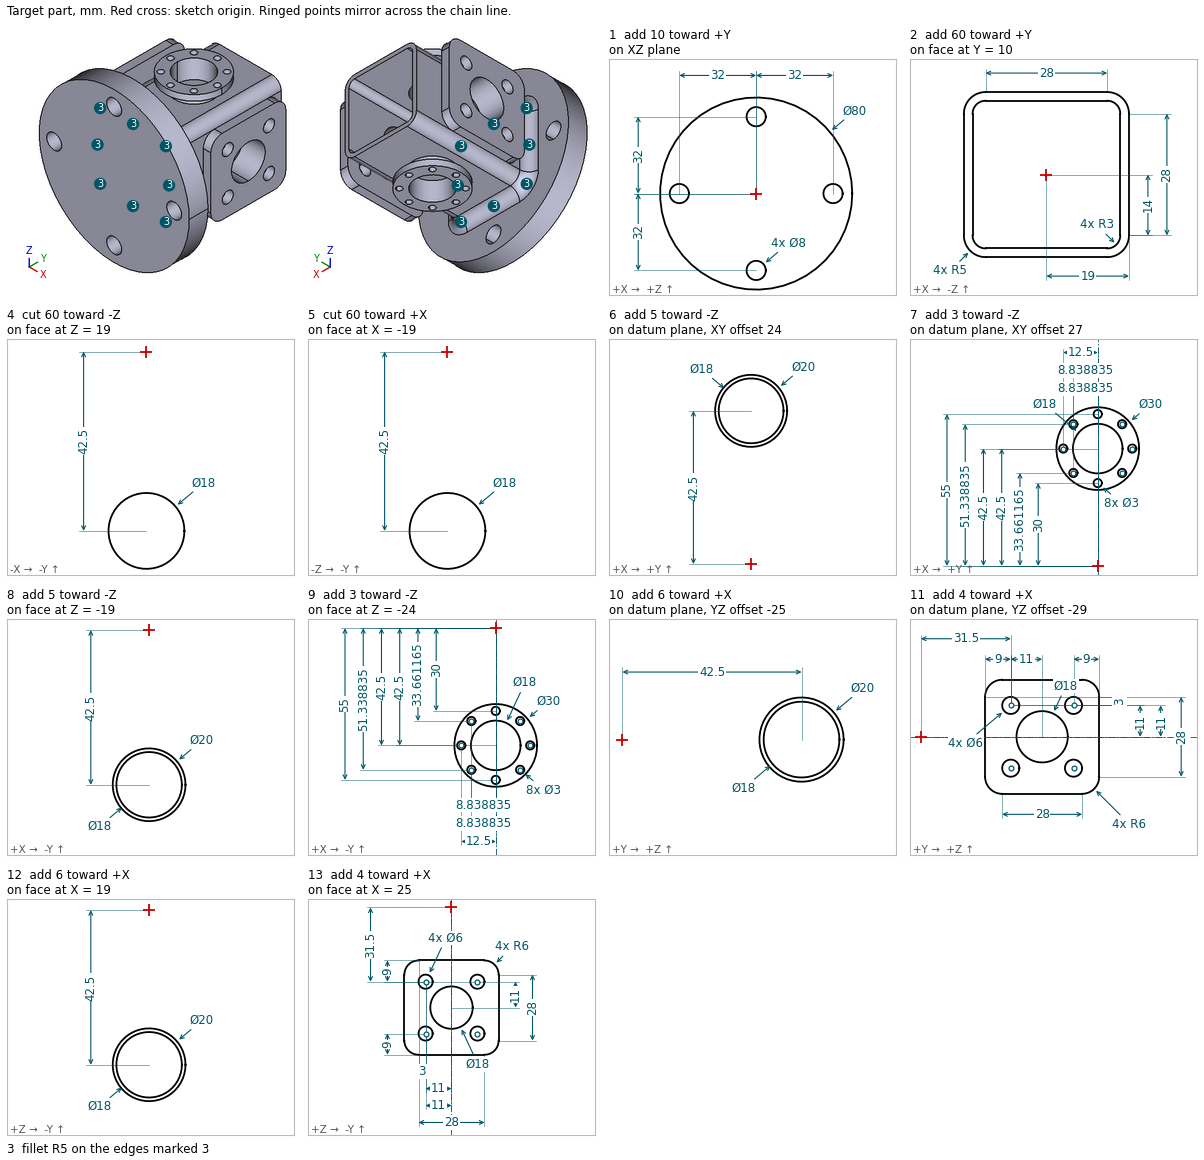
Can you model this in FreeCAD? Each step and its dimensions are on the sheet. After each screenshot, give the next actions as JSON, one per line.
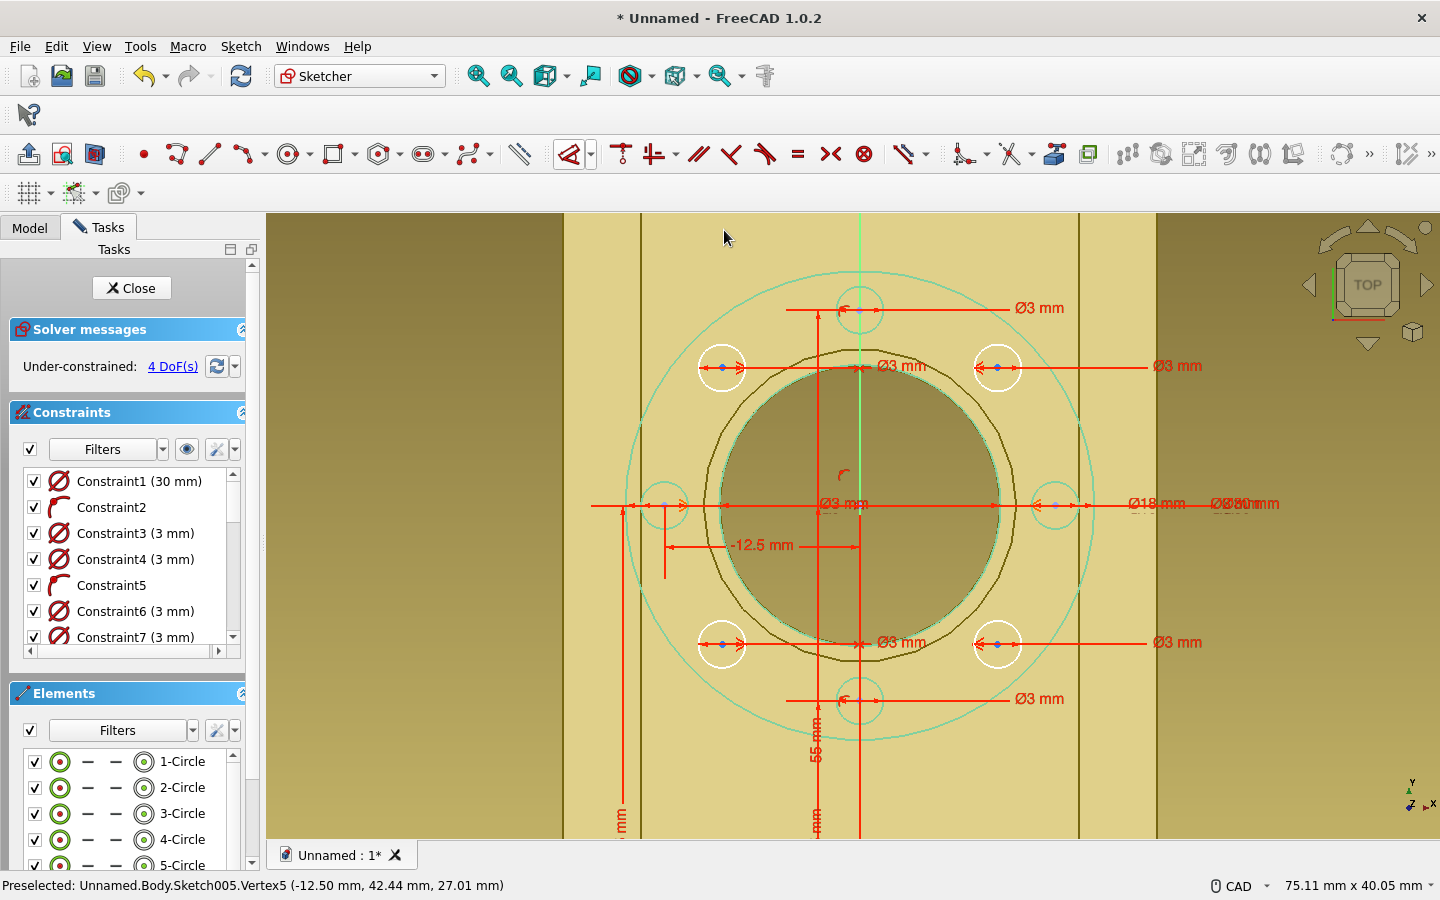
{"action": "left_click", "coordinate": [722, 644]}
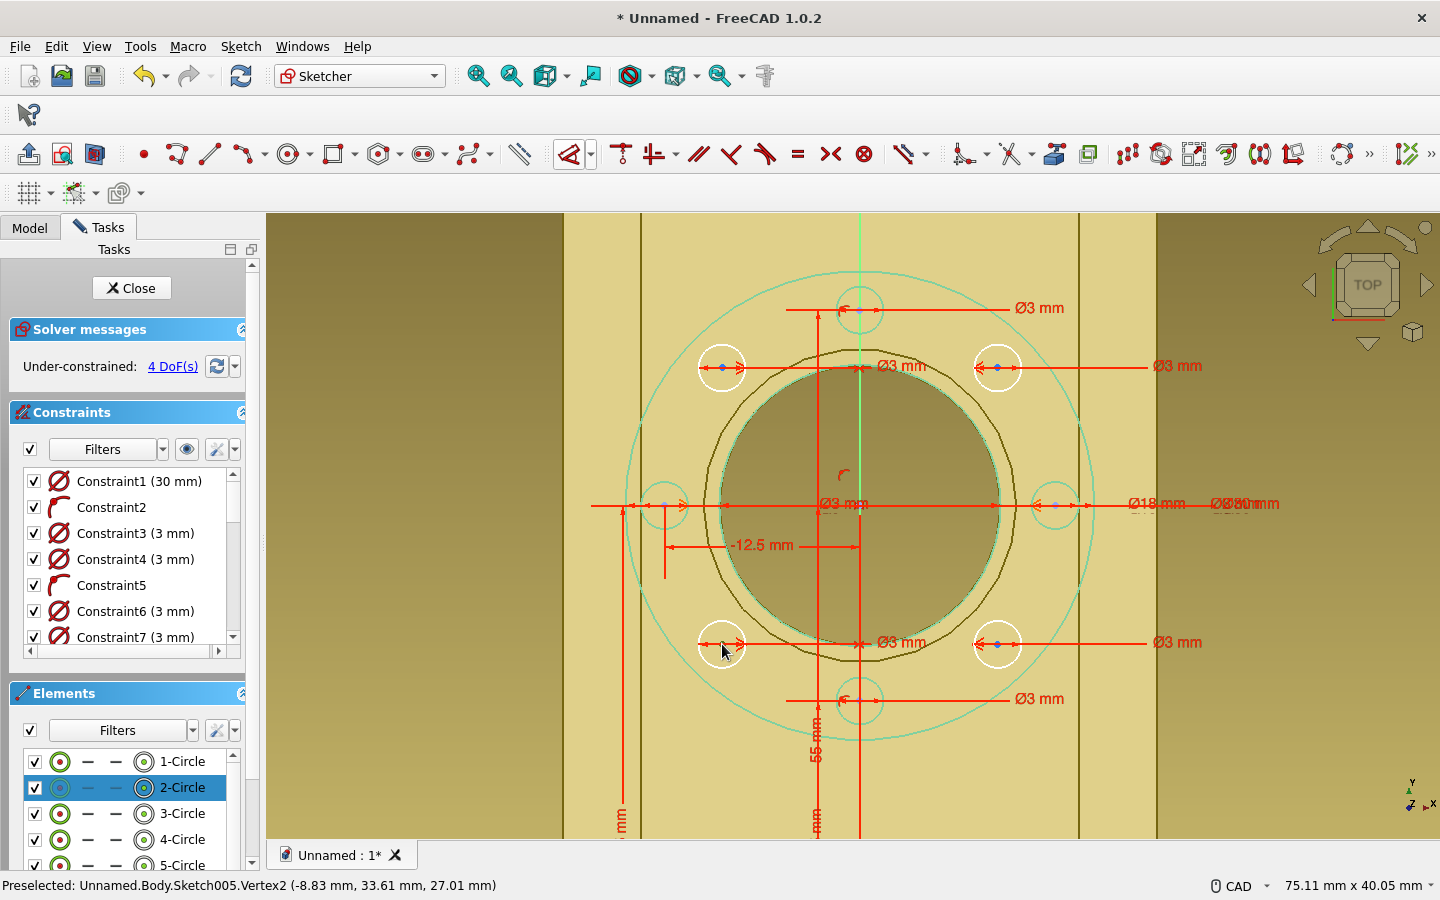
{"action": "key", "text": "l"}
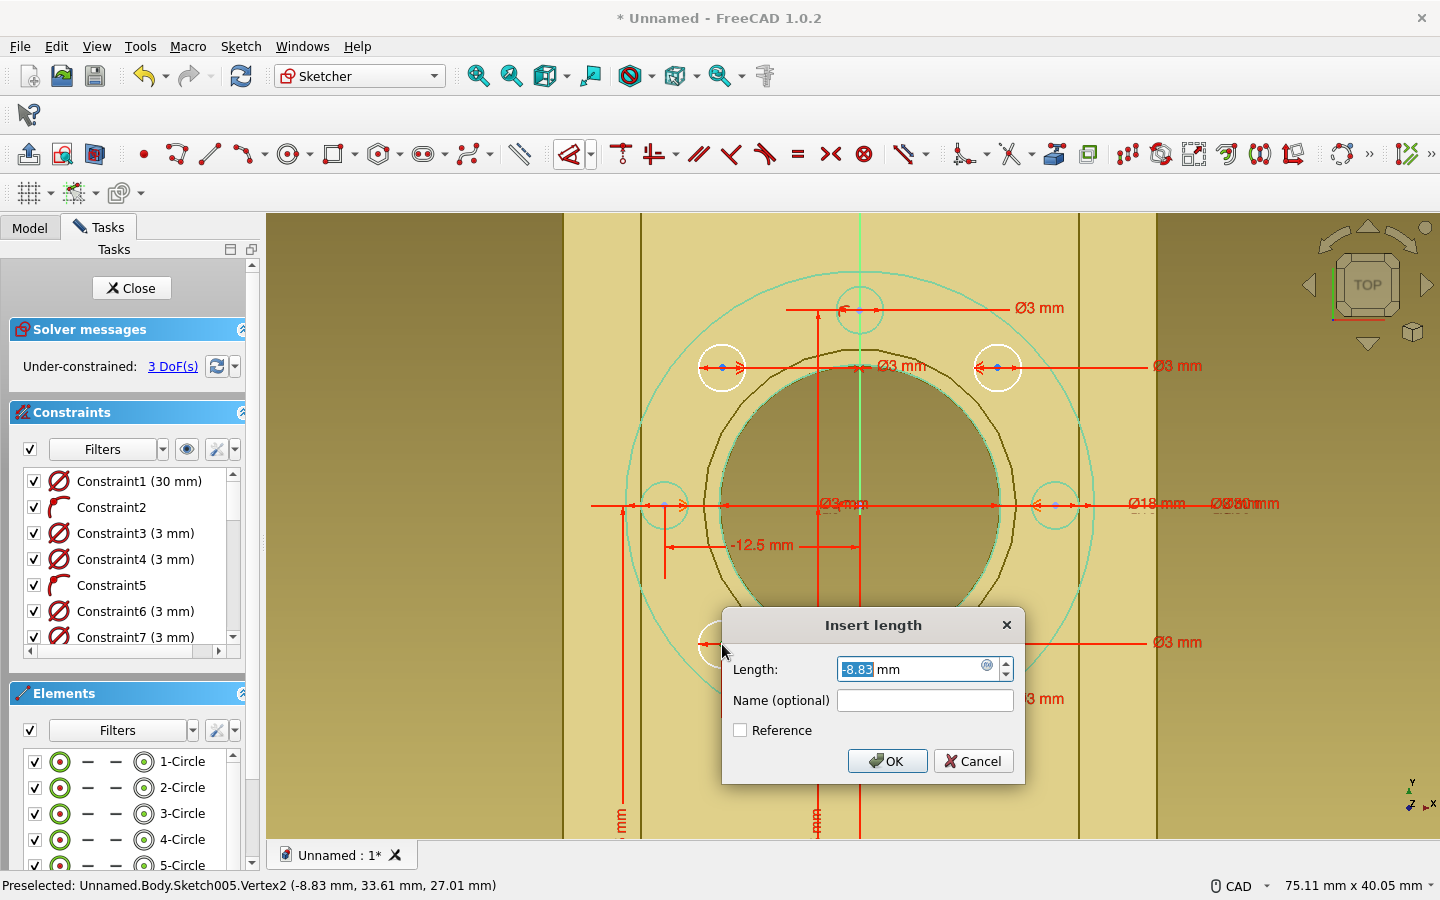
{"action": "type", "text": "-8.838835"}
{"action": "key", "text": "Return"}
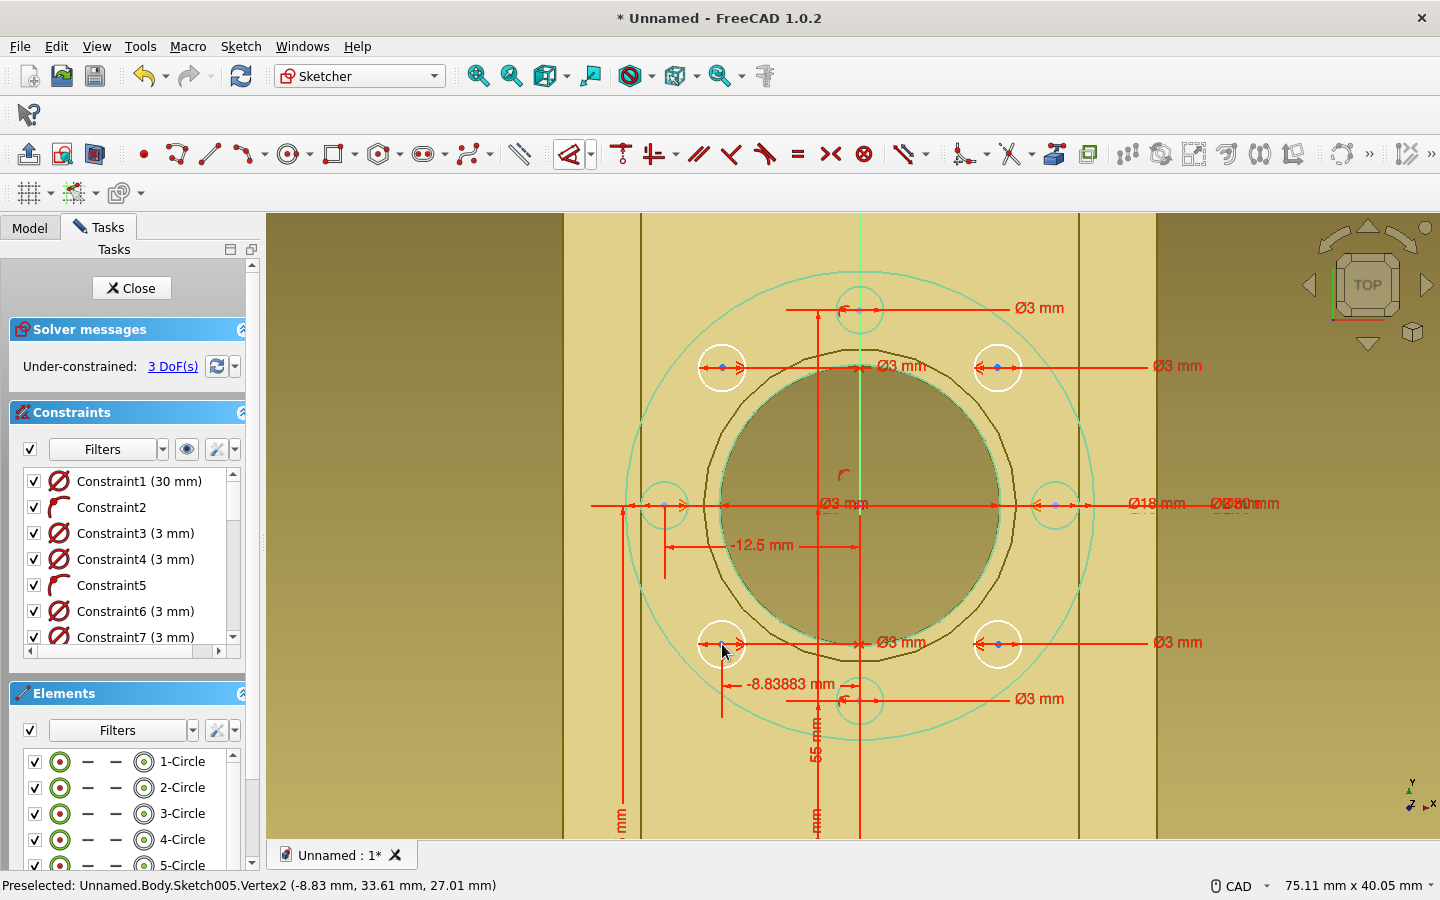
{"action": "left_click", "coordinate": [722, 368]}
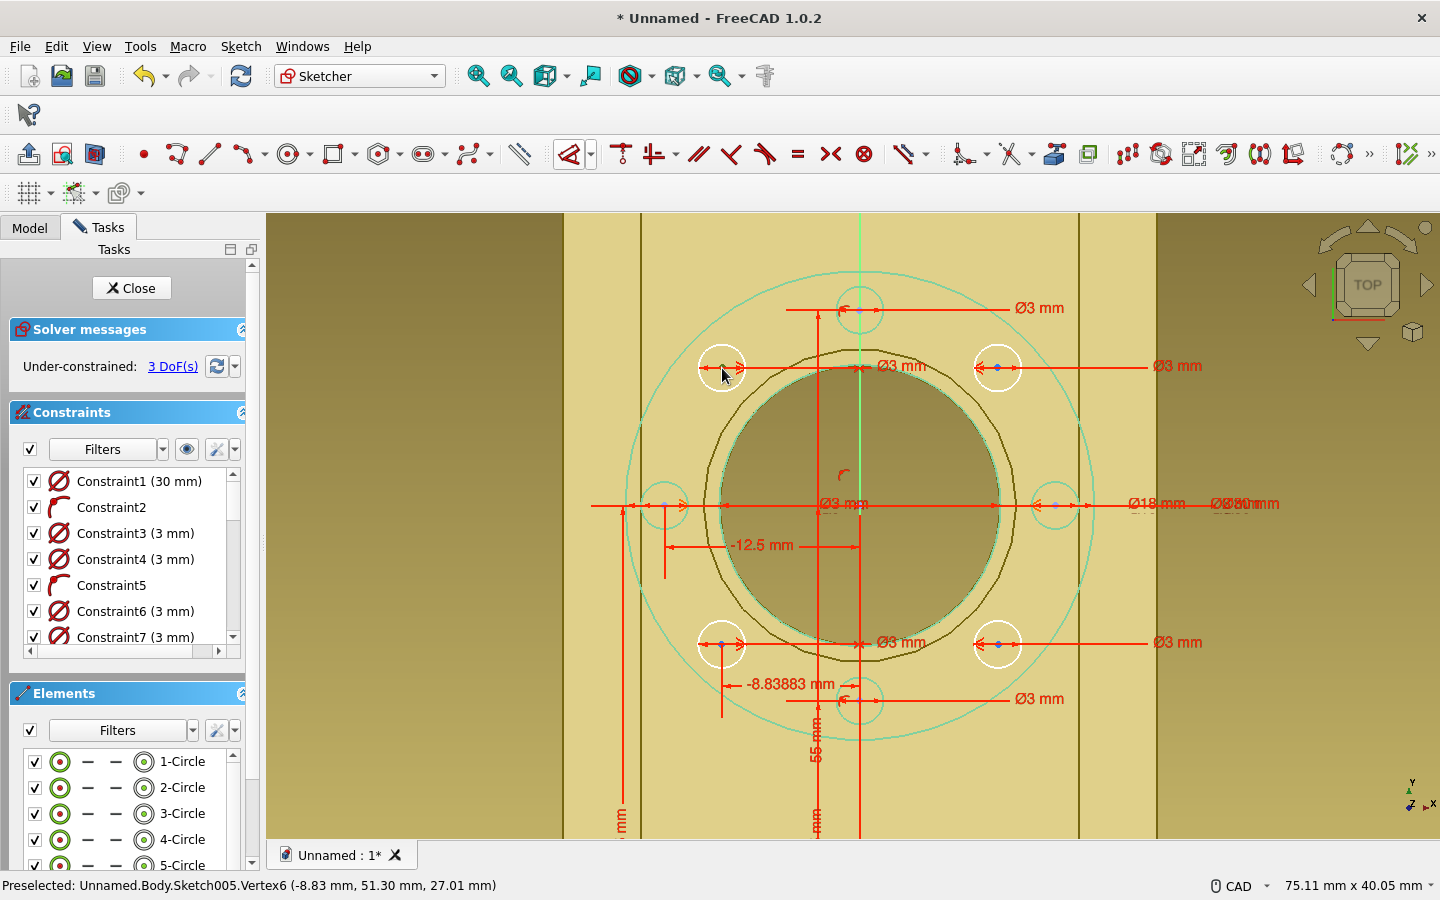
{"action": "left_click", "coordinate": [590, 154]}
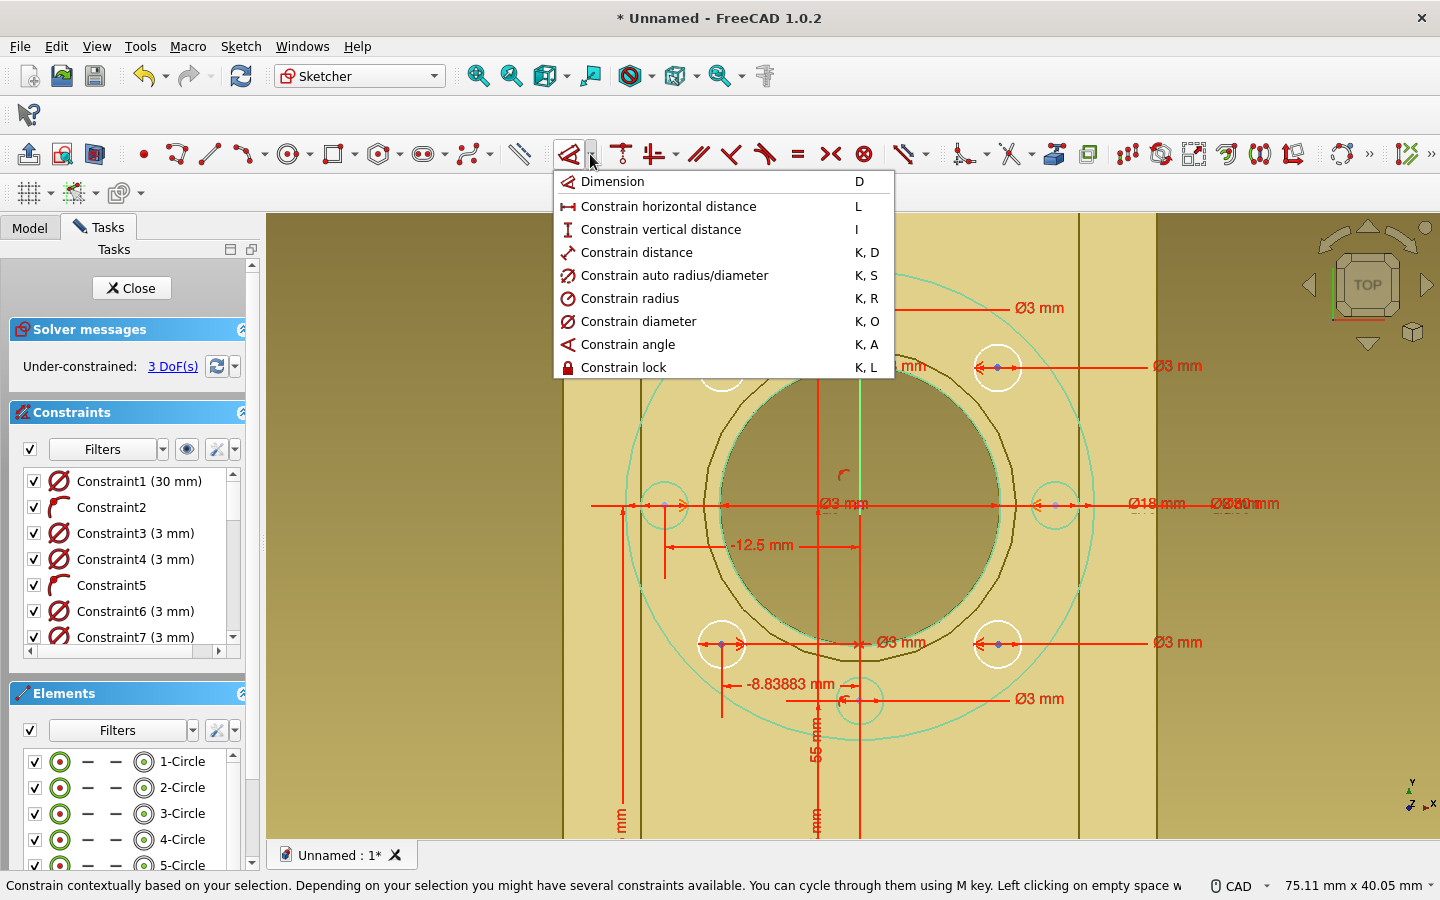
{"action": "left_click", "coordinate": [724, 206]}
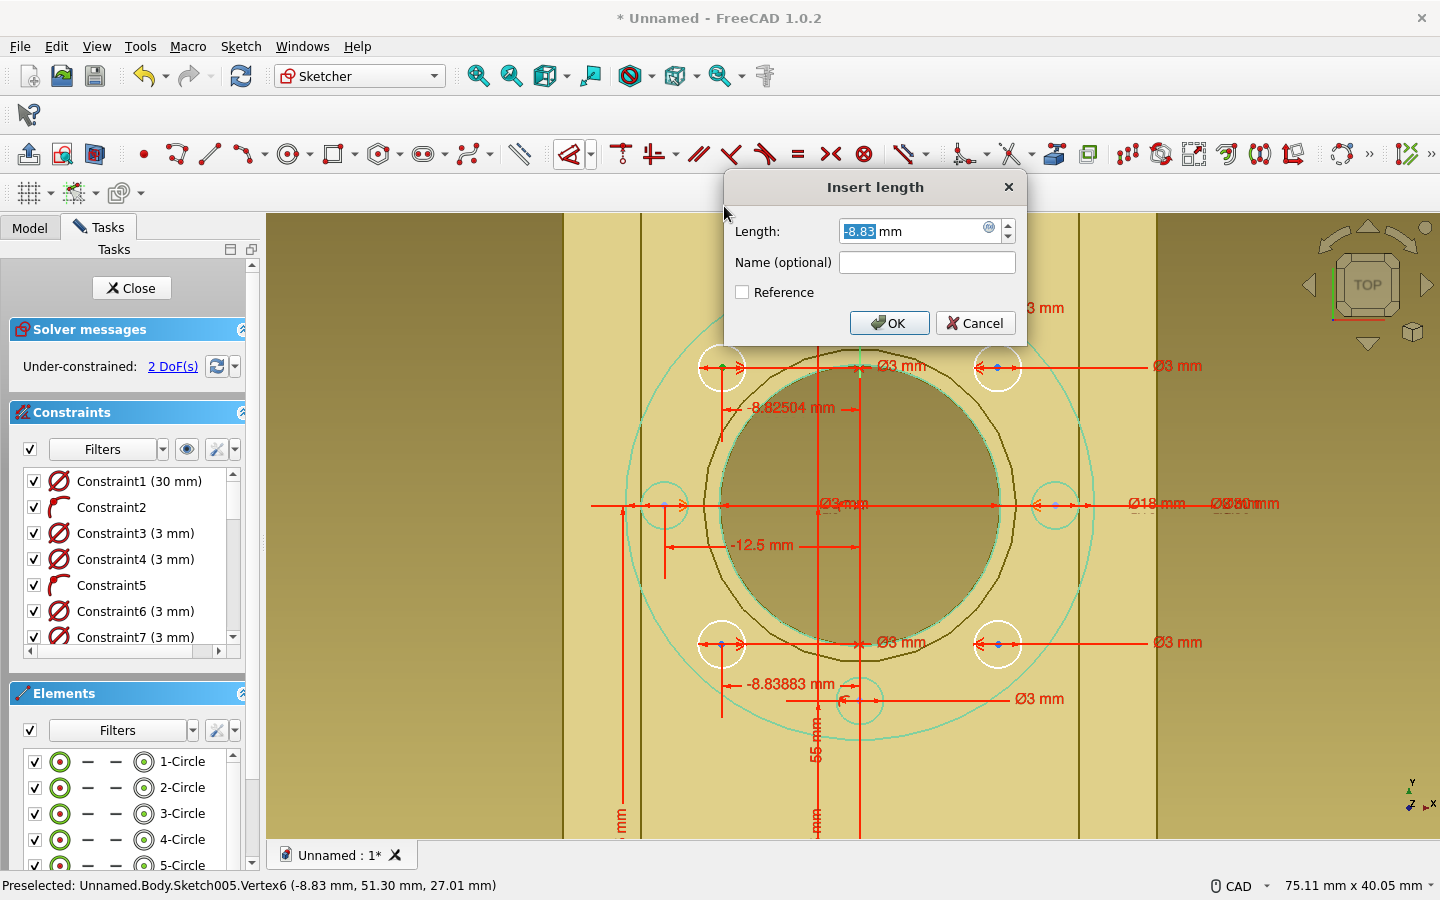
{"action": "type", "text": "-8.838835"}
{"action": "key", "text": "Return"}